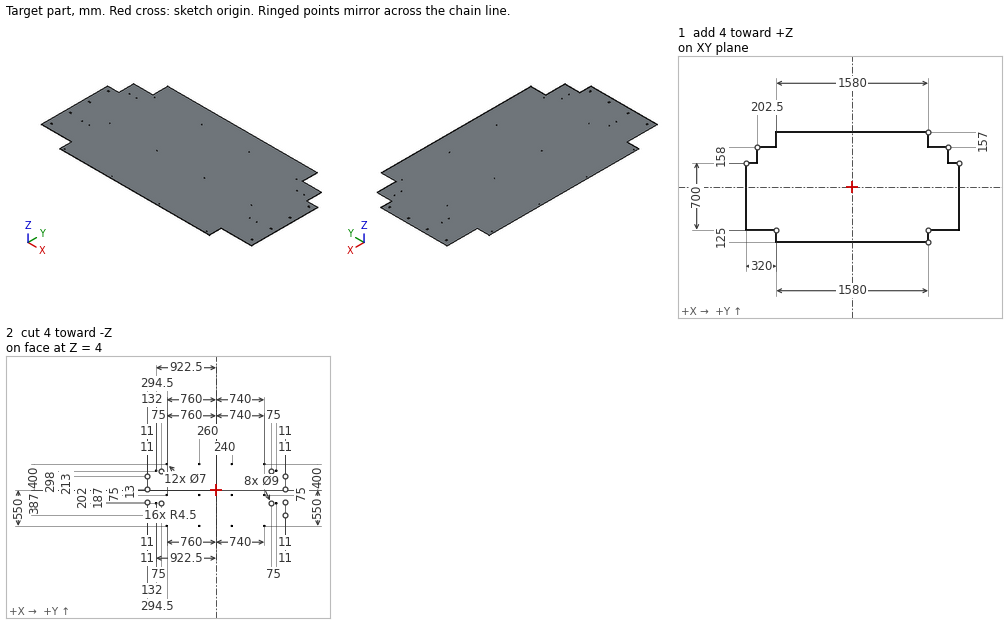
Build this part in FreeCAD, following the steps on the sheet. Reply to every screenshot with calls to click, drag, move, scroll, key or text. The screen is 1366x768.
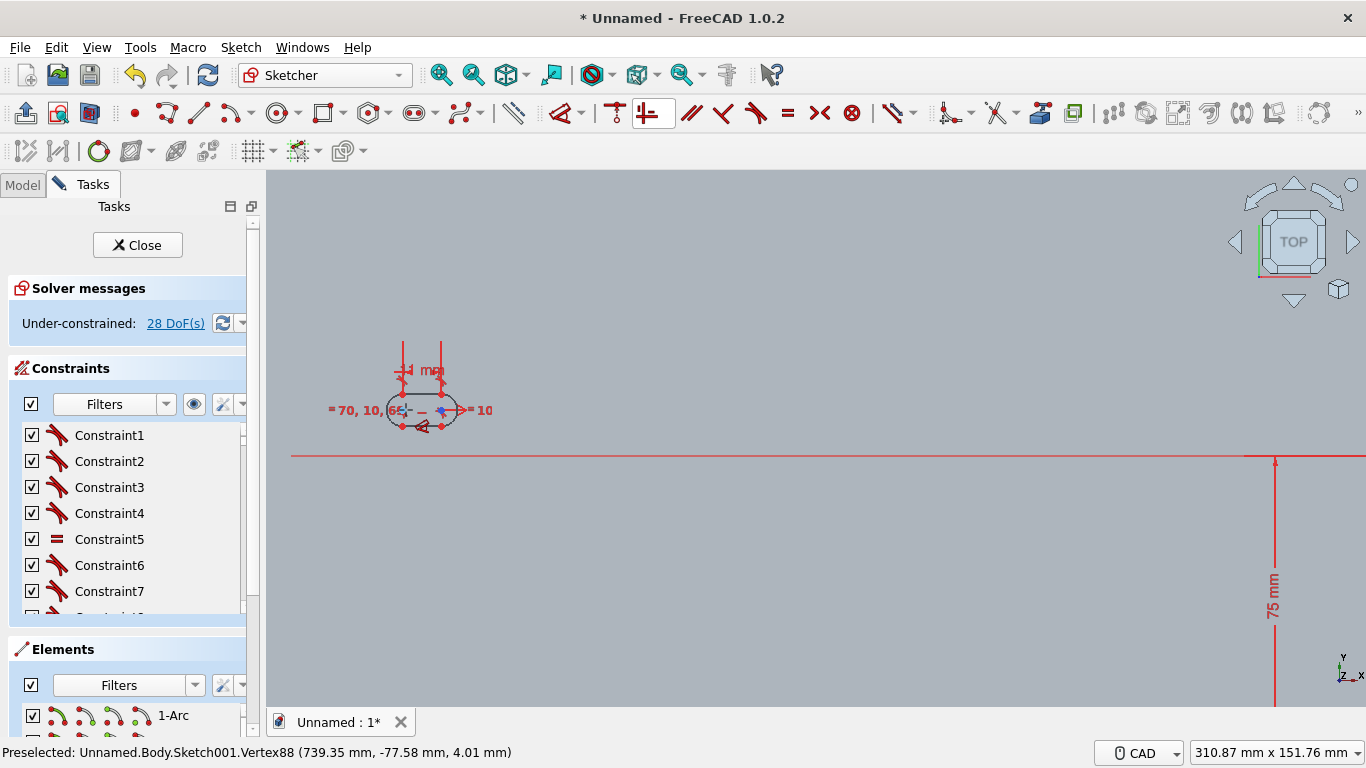
click(403, 410)
click(369, 433)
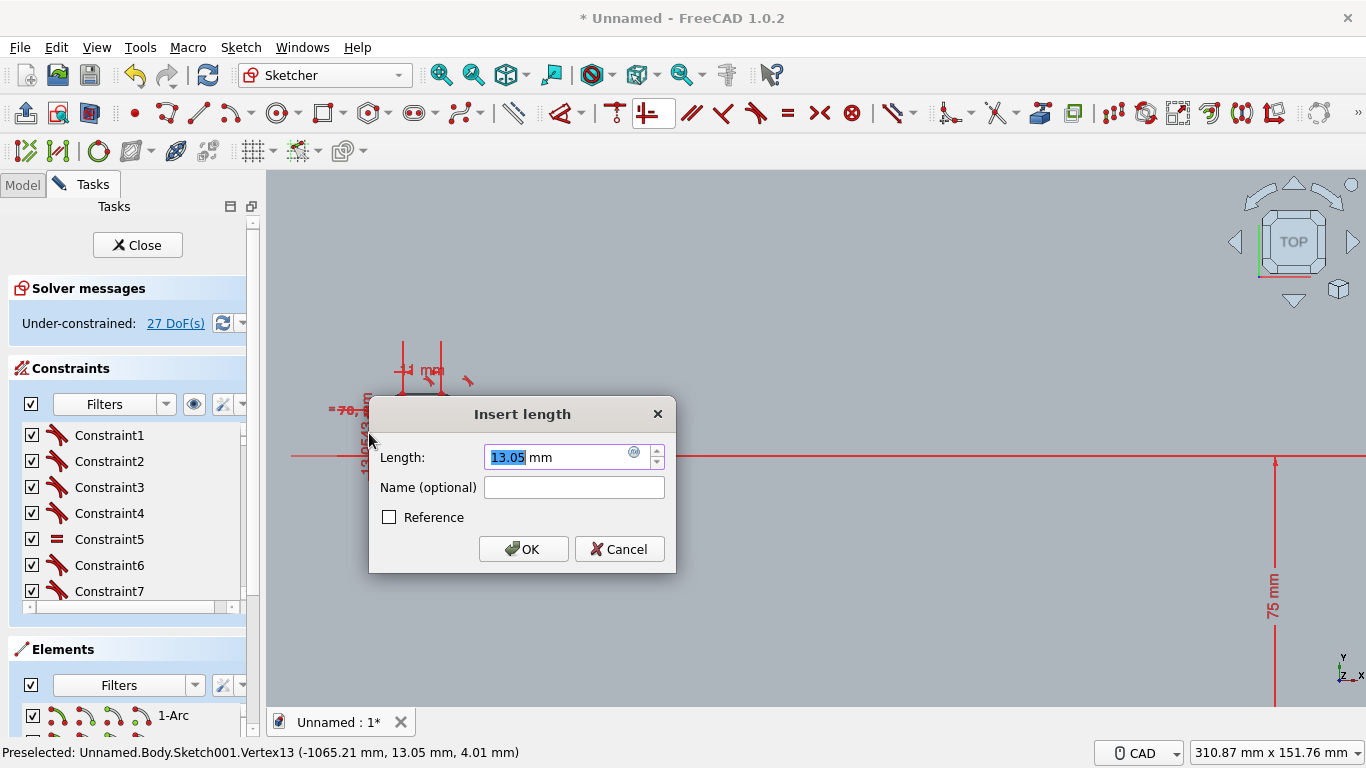
text(13)
key(Return)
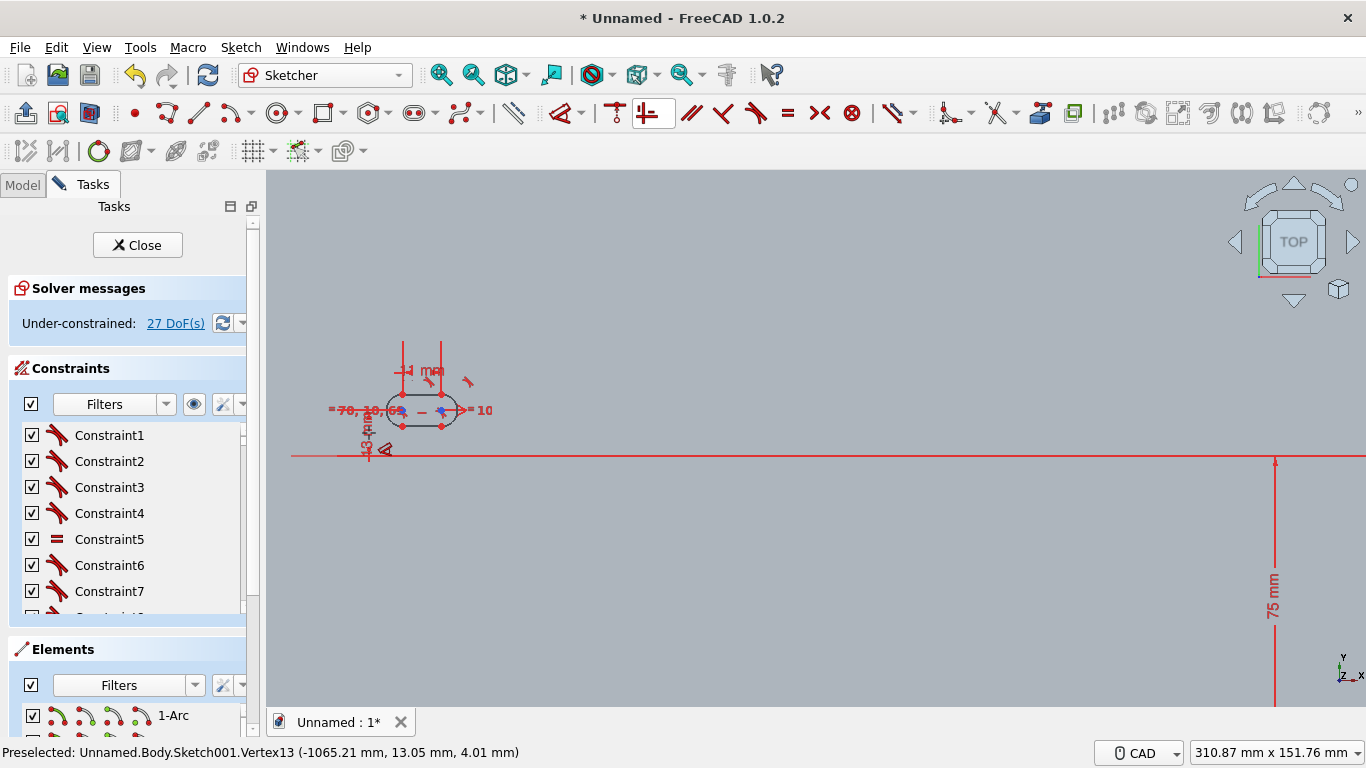
scroll(406, 410, down, 12)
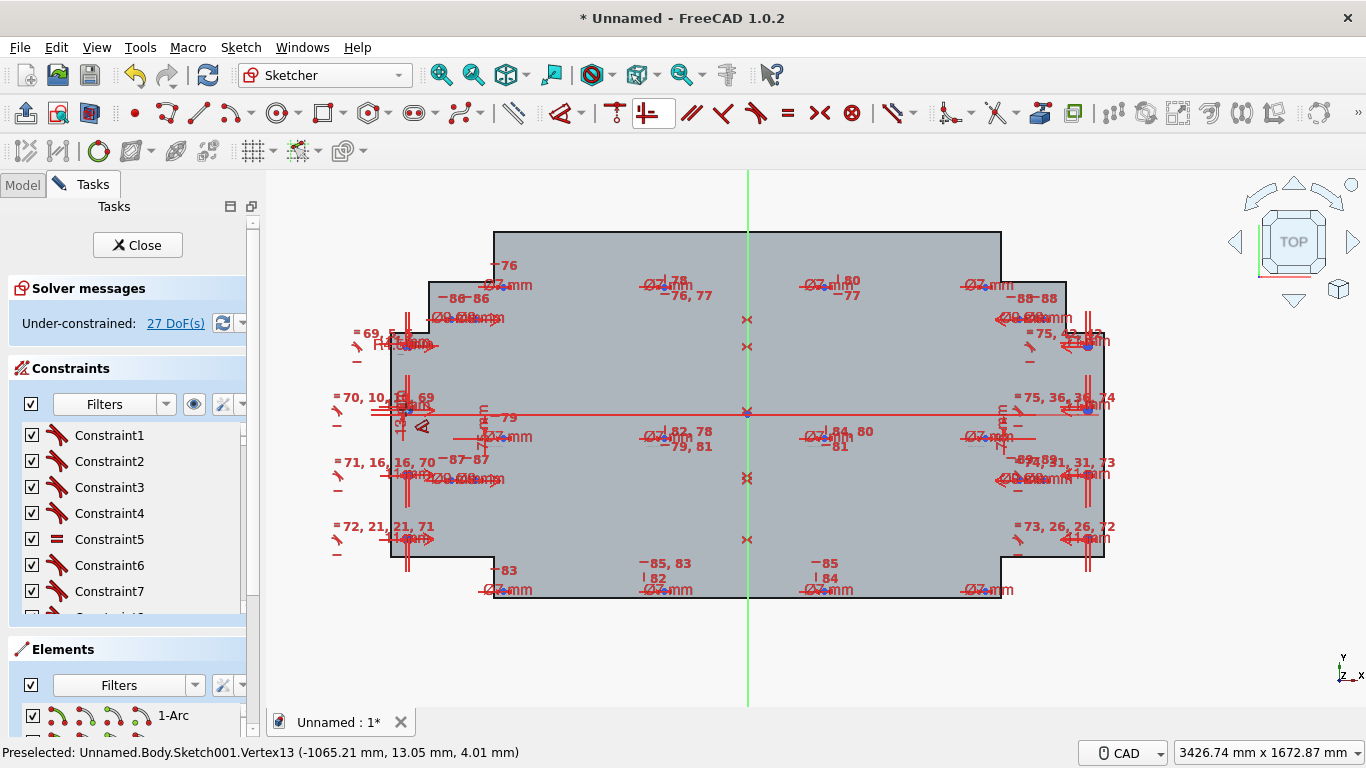
click(504, 287)
click(626, 253)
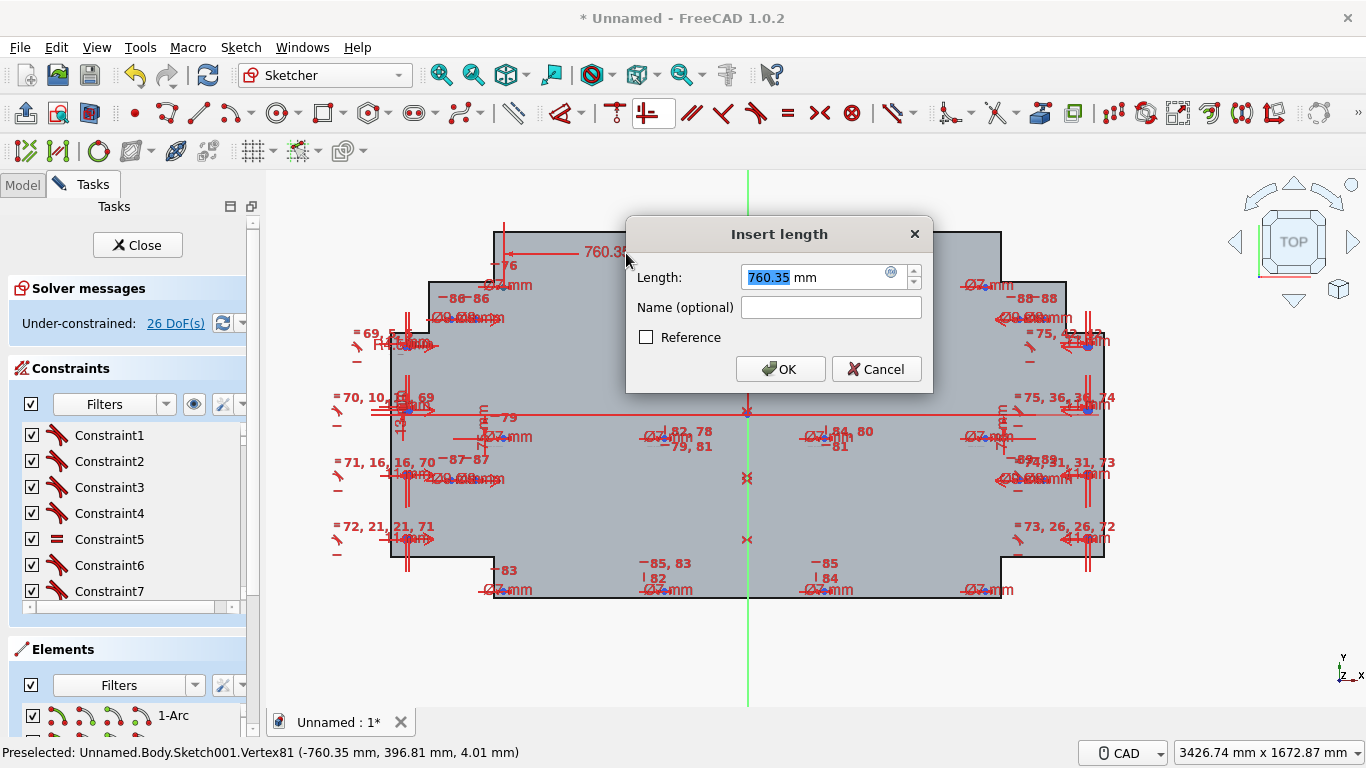
text(760)
key(Return)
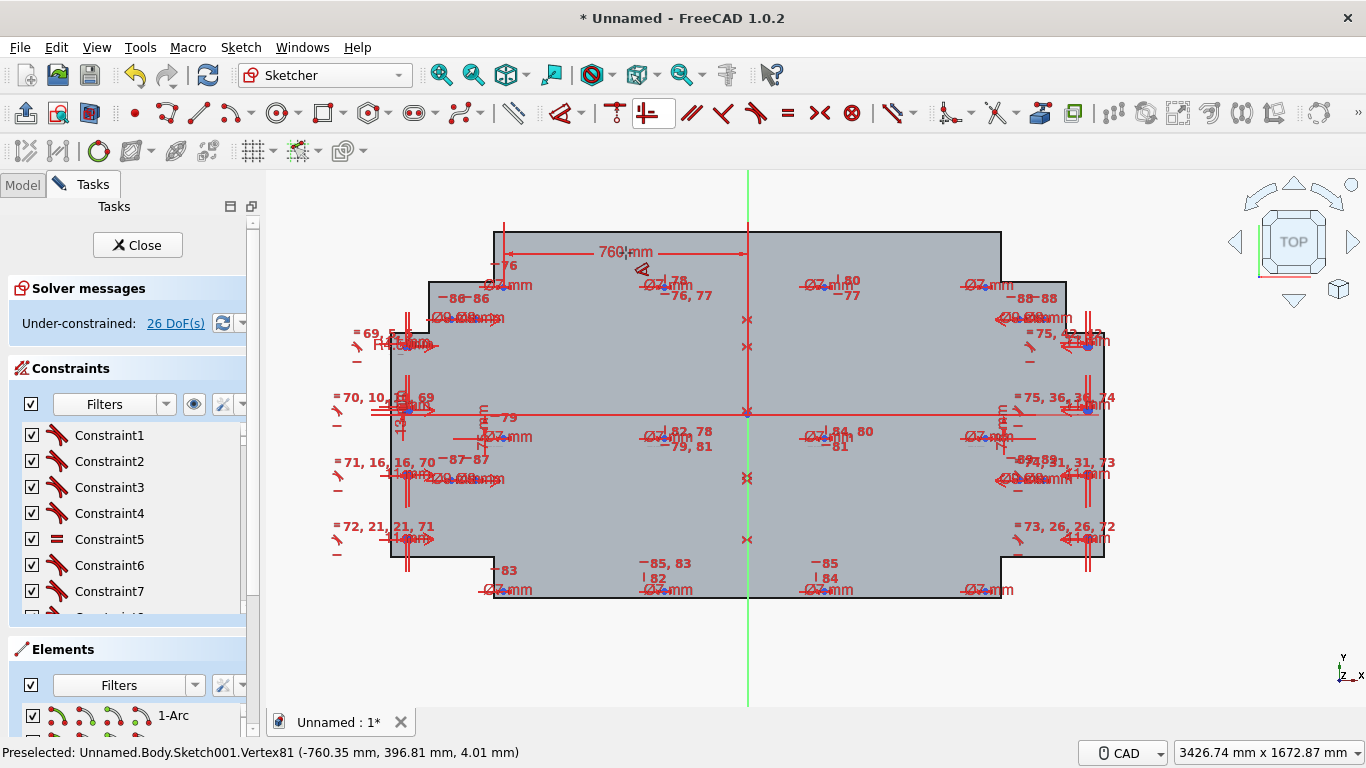
click(504, 287)
click(470, 380)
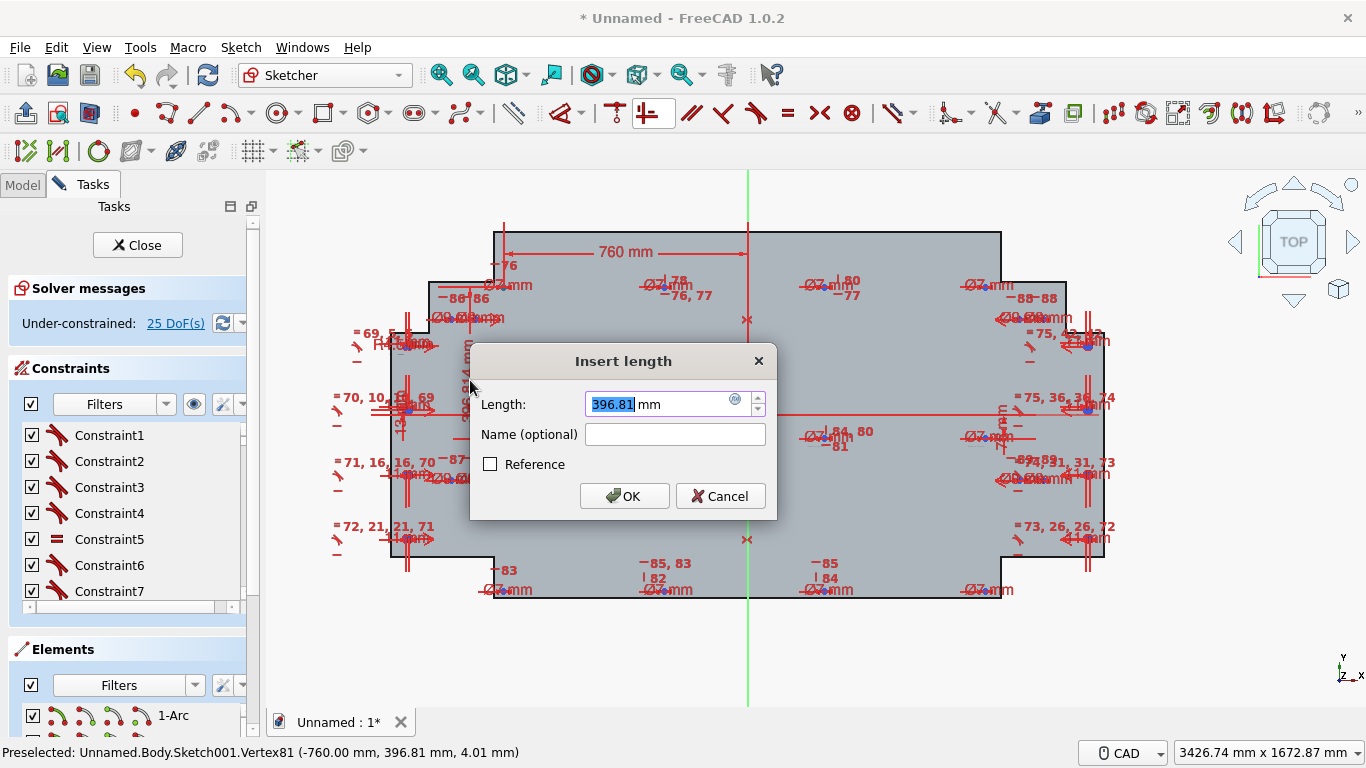
text(400)
key(Return)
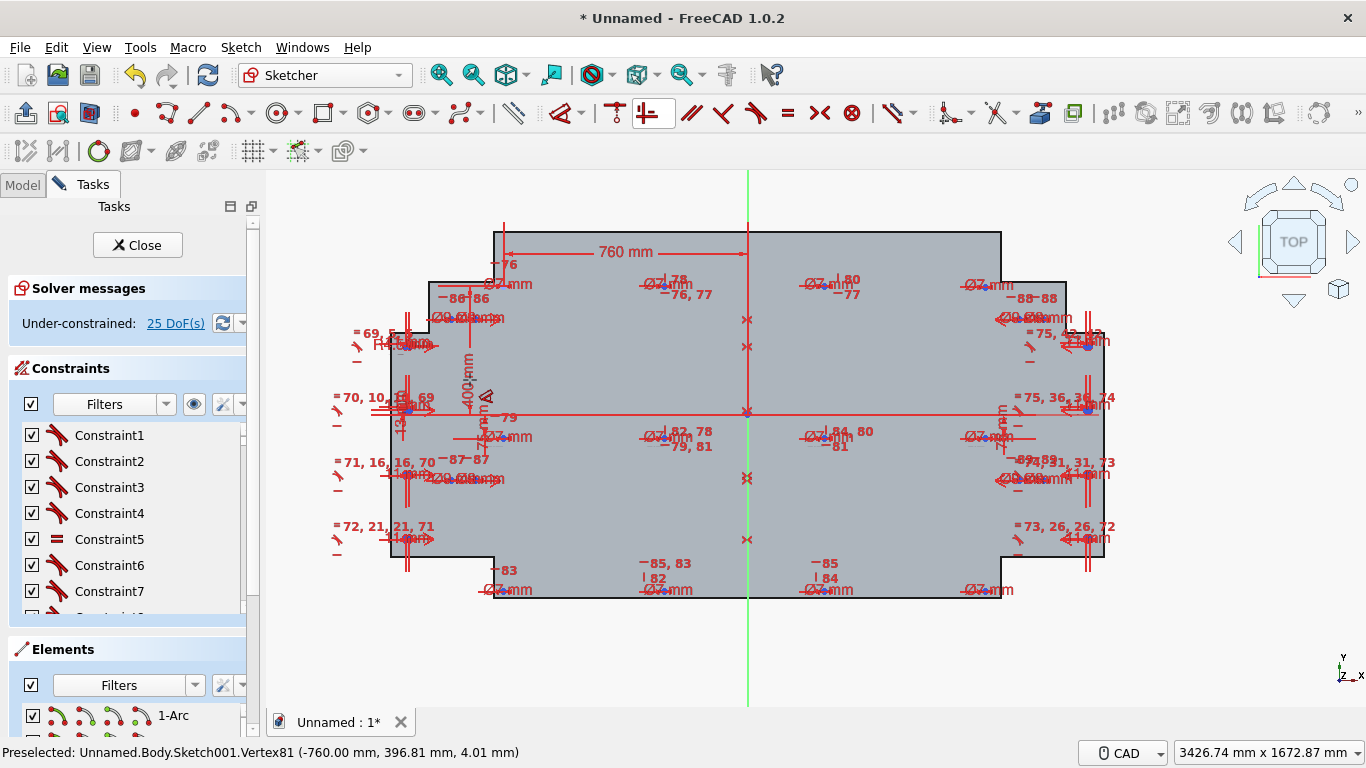
click(664, 286)
click(706, 252)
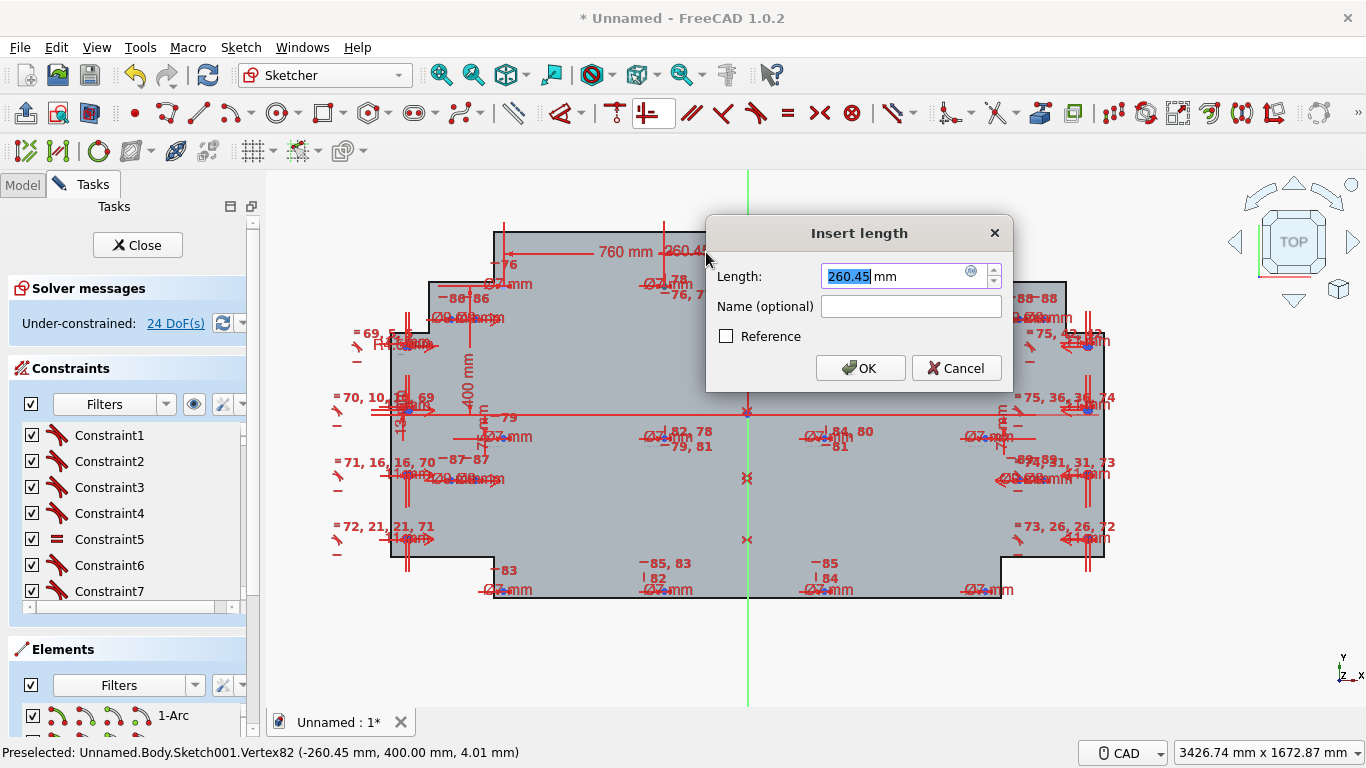
text(260)
key(Return)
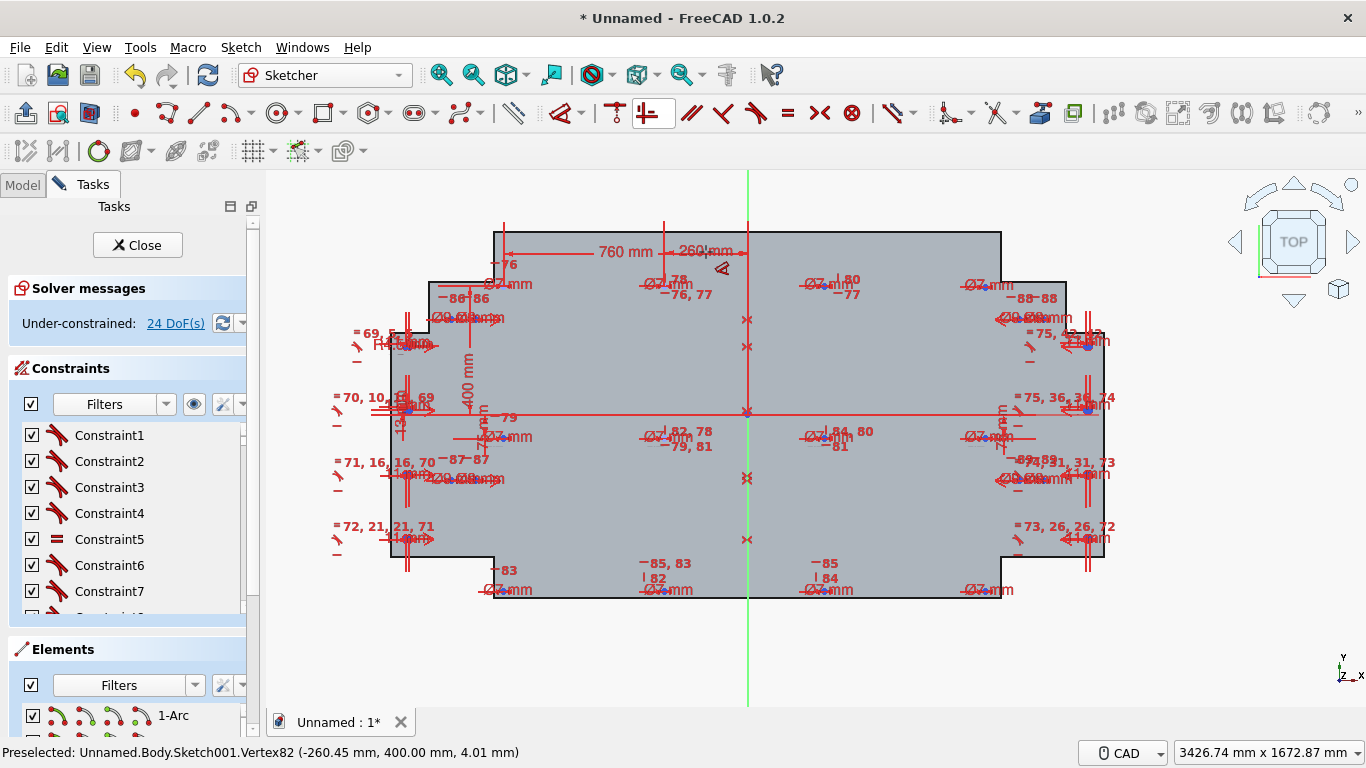
click(825, 286)
click(786, 252)